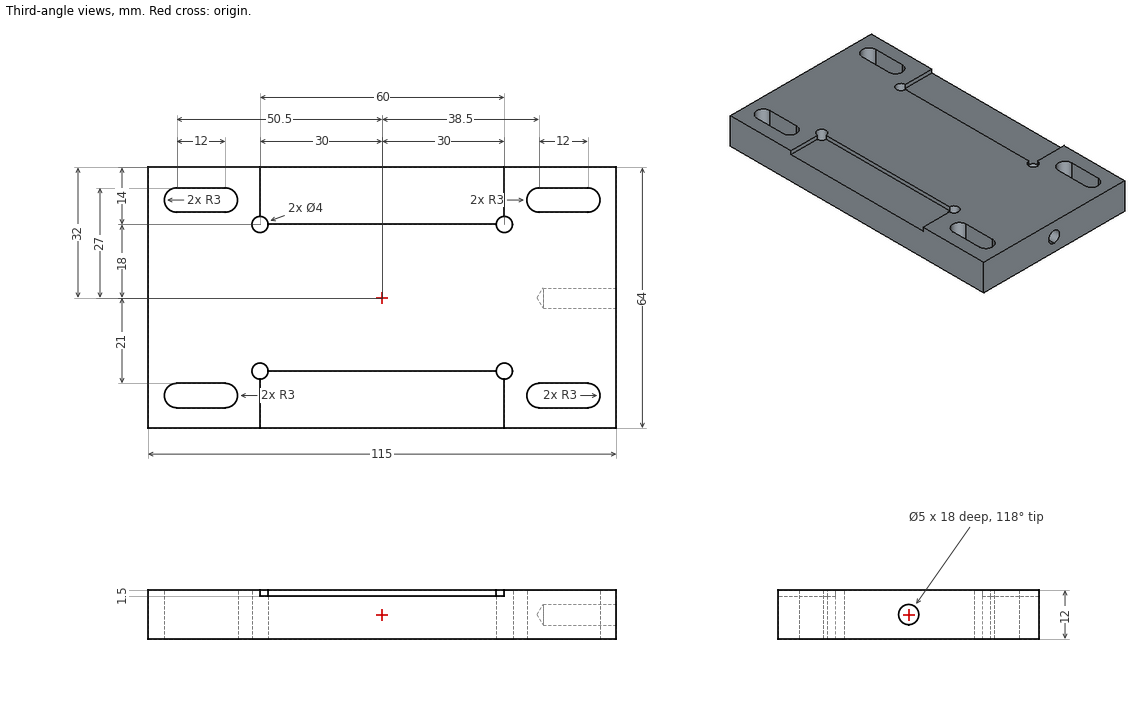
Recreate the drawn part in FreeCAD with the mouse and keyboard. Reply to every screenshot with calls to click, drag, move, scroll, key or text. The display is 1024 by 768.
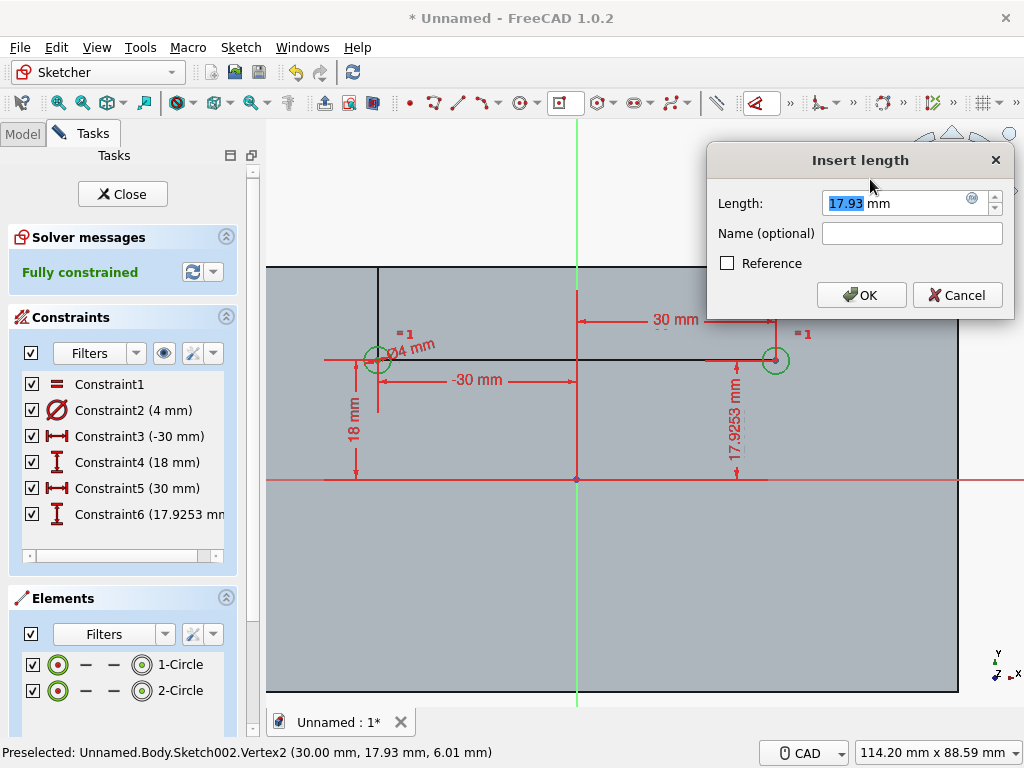
text(18)
key(Return)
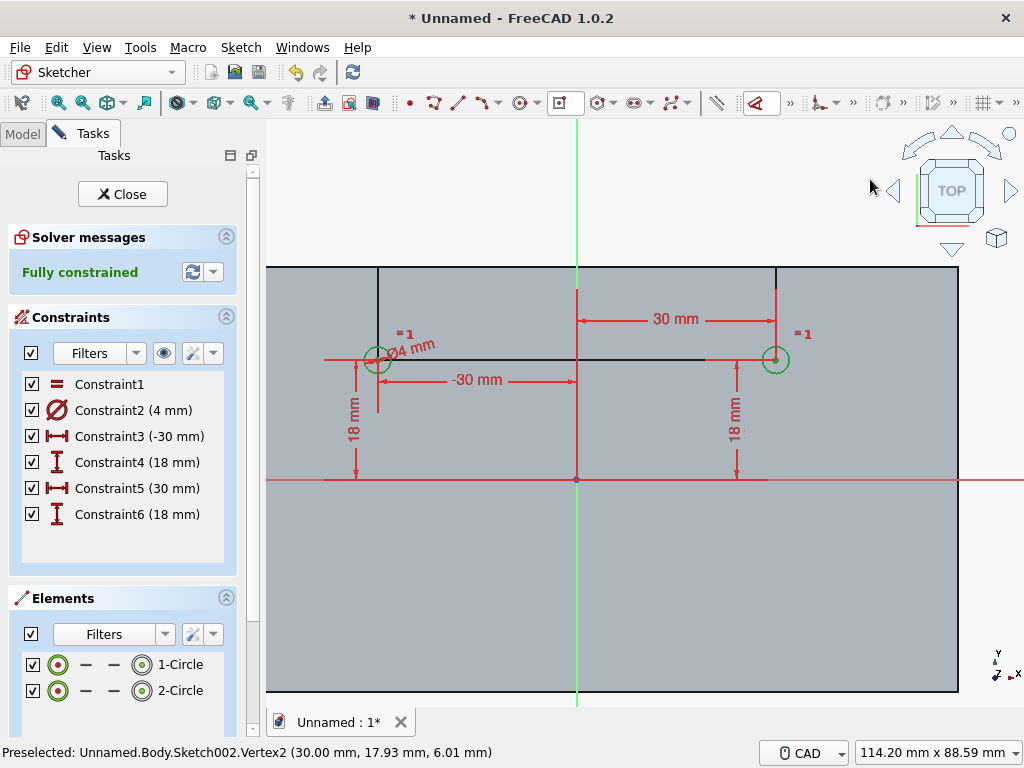
click(123, 194)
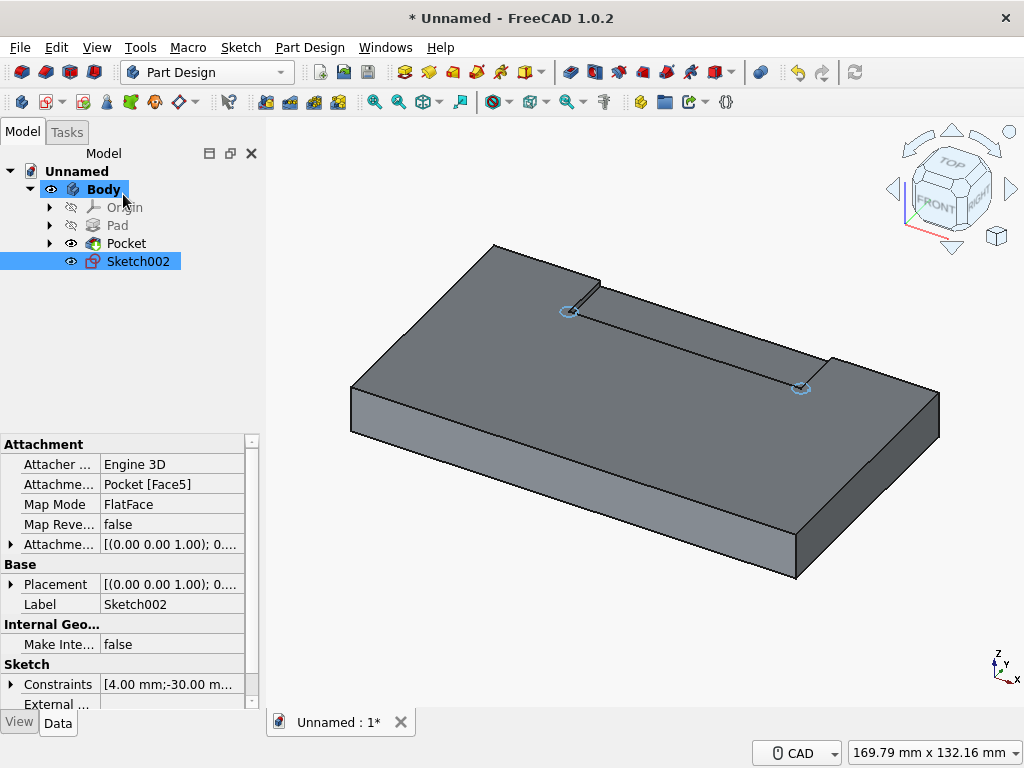
click(572, 72)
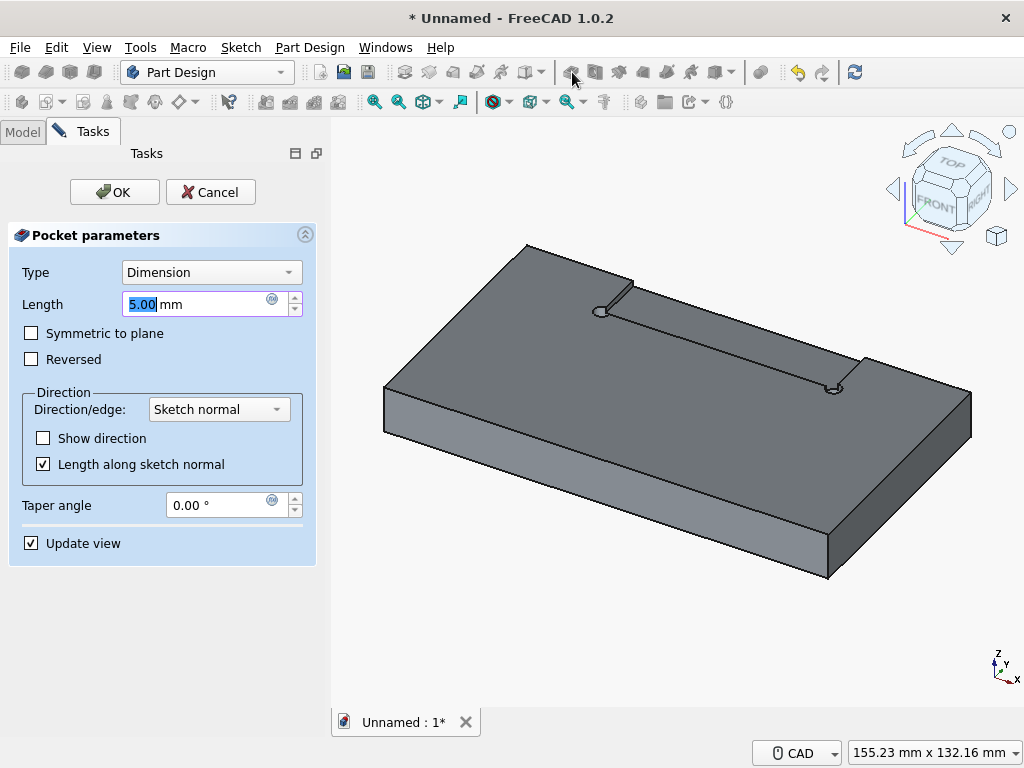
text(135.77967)
key(Tab)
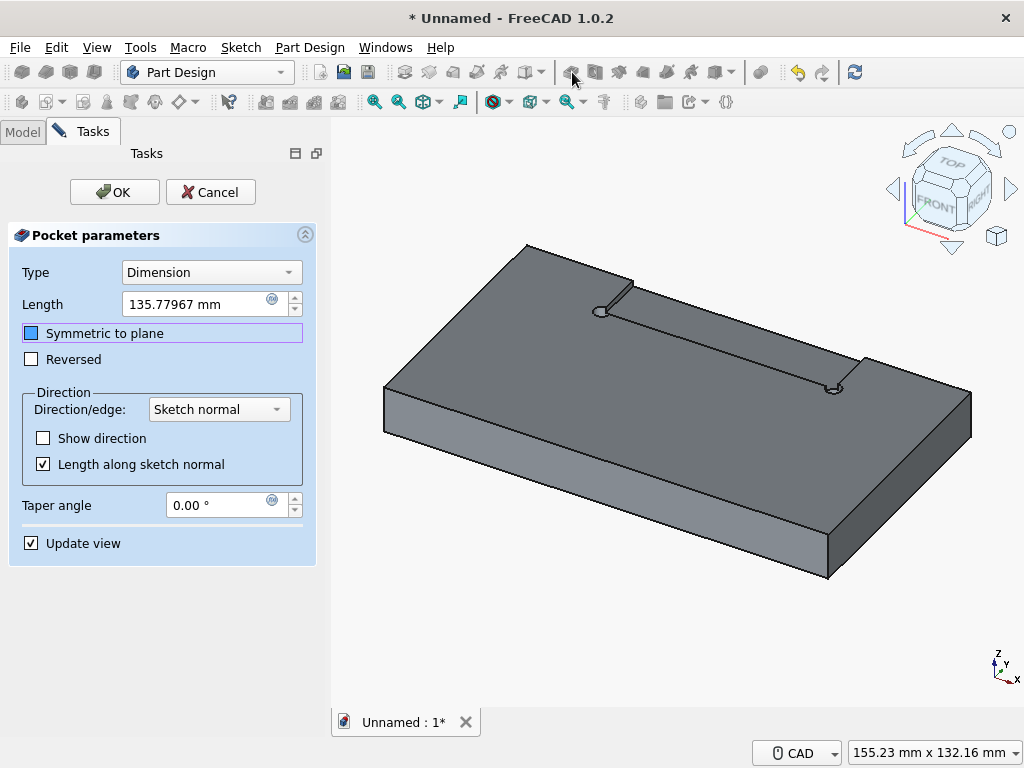
click(30, 333)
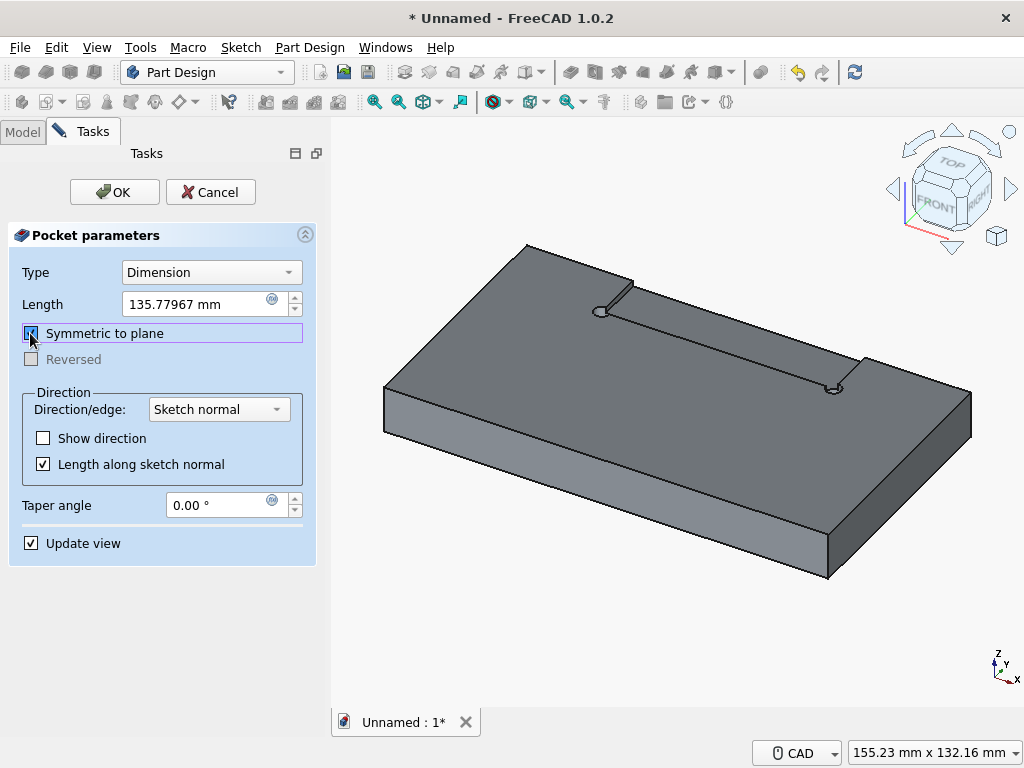
click(115, 192)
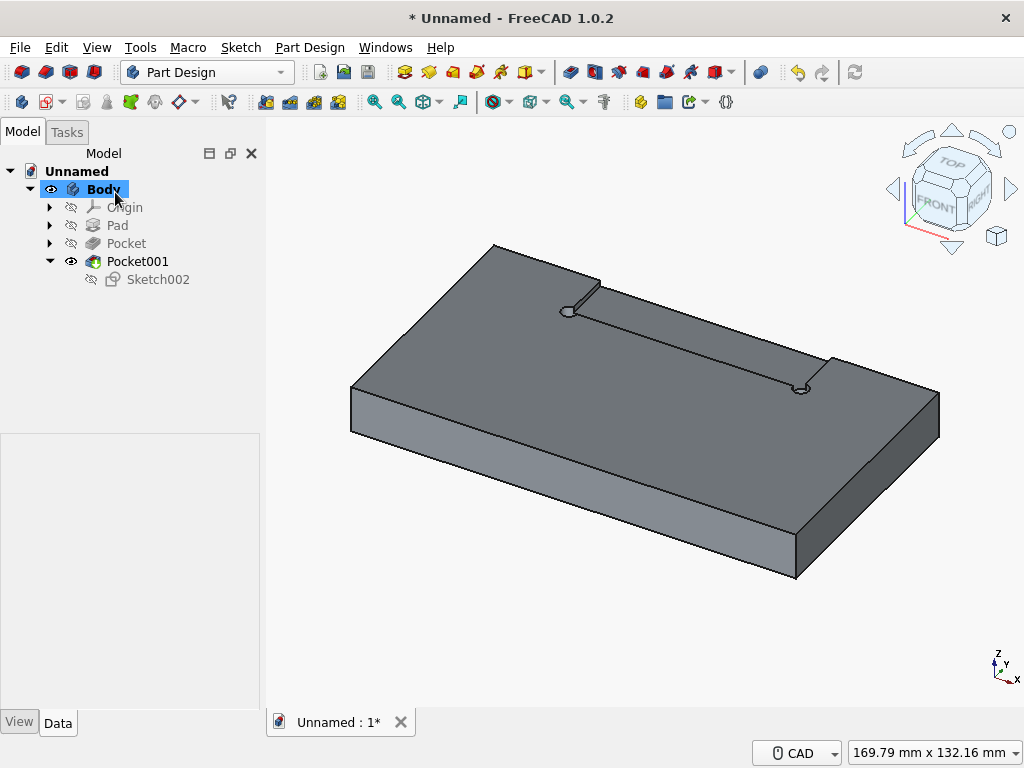
click(116, 243)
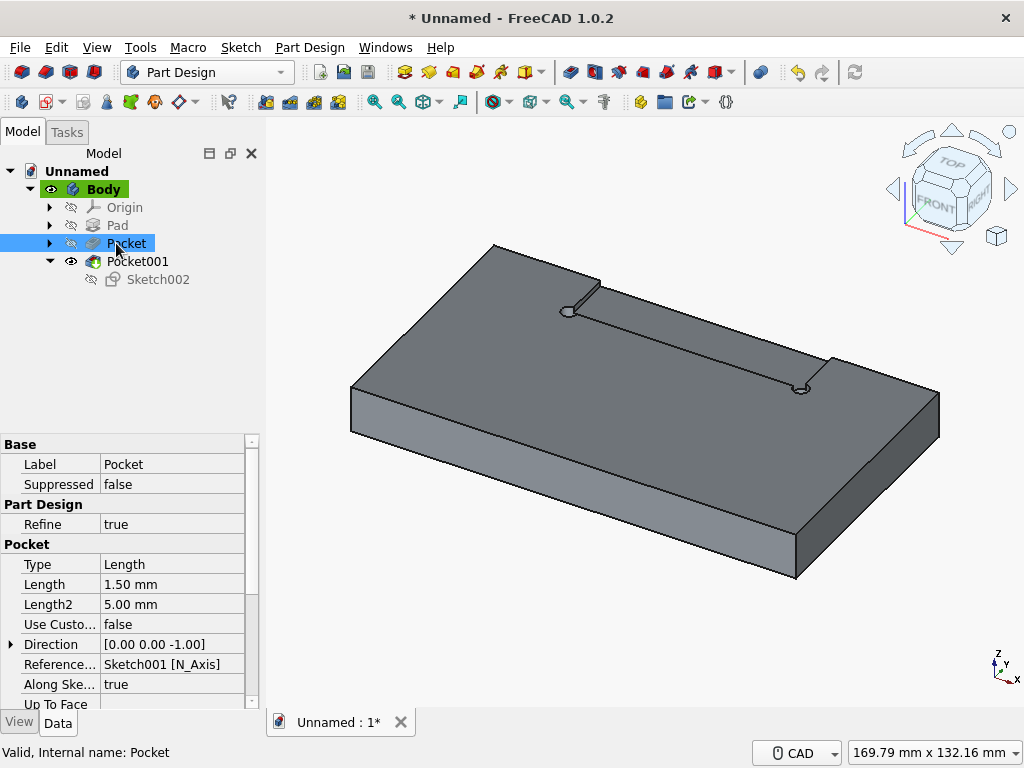
click(116, 261, ctrl)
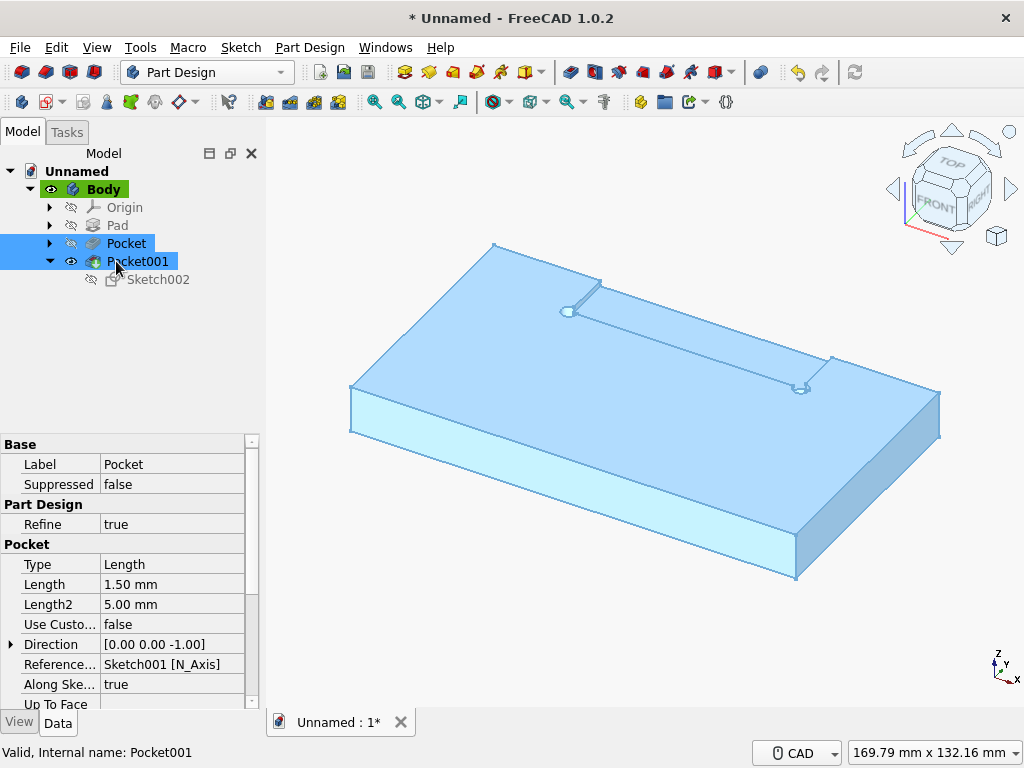
click(266, 102)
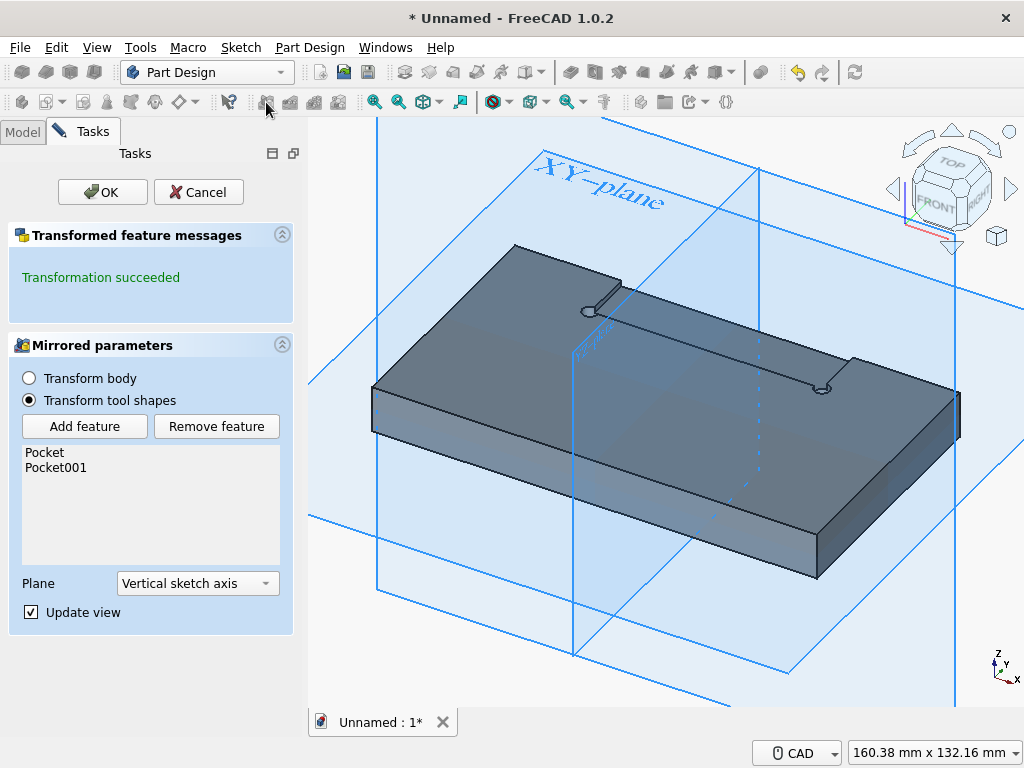
click(198, 584)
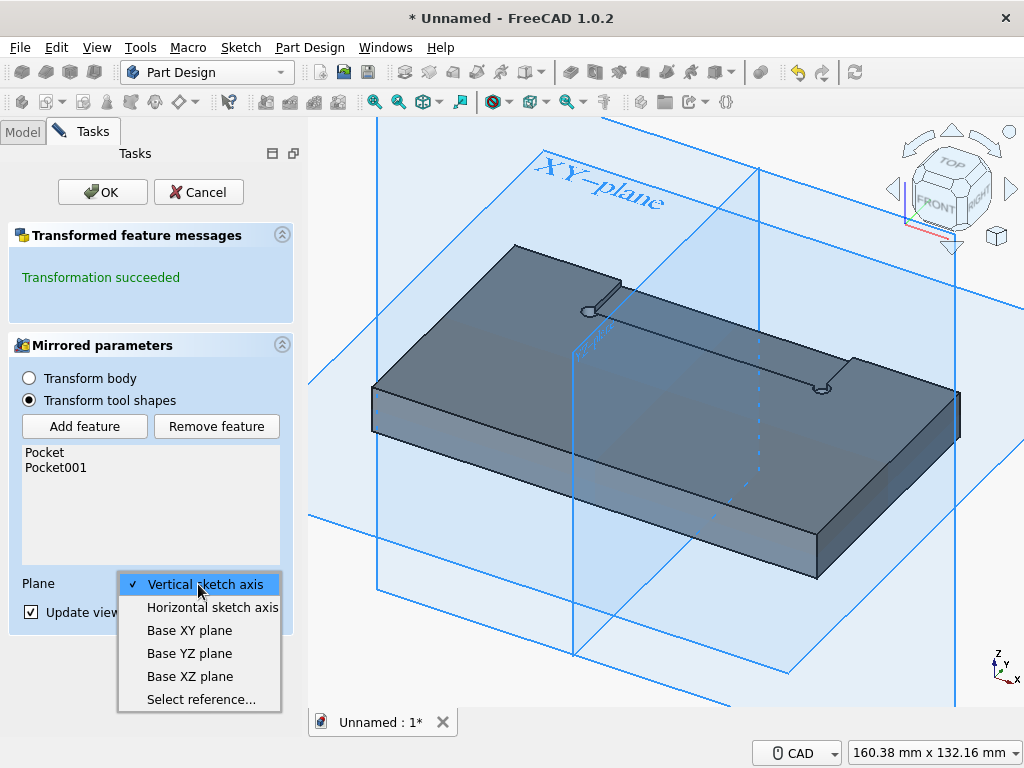
click(198, 676)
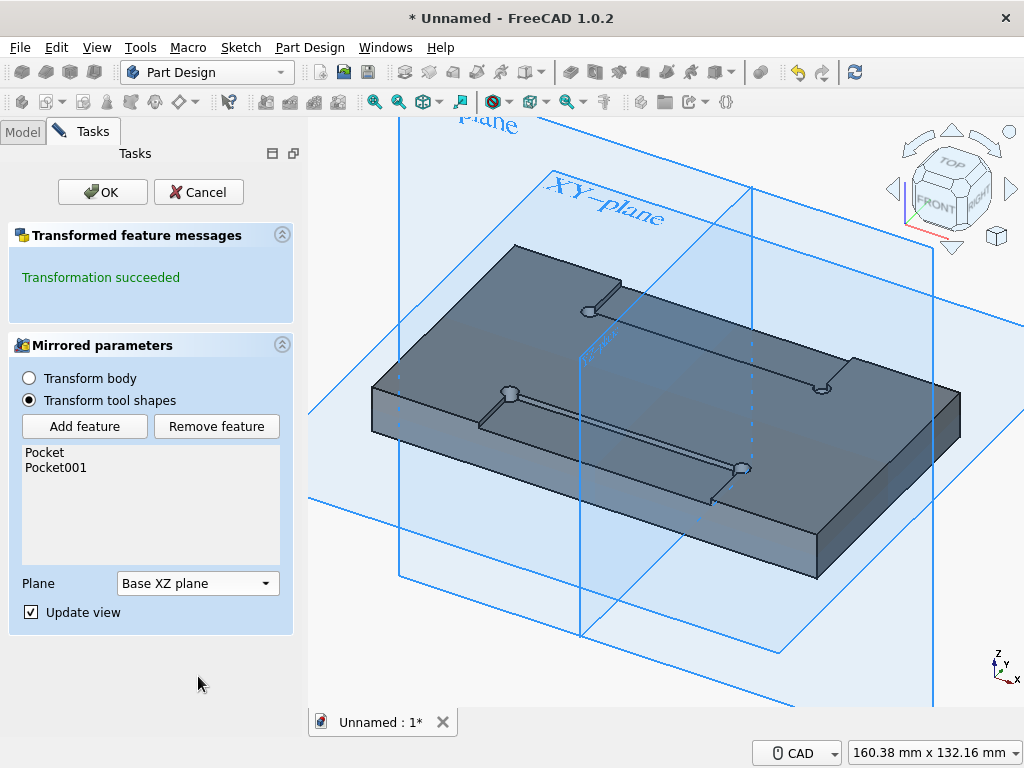
click(103, 192)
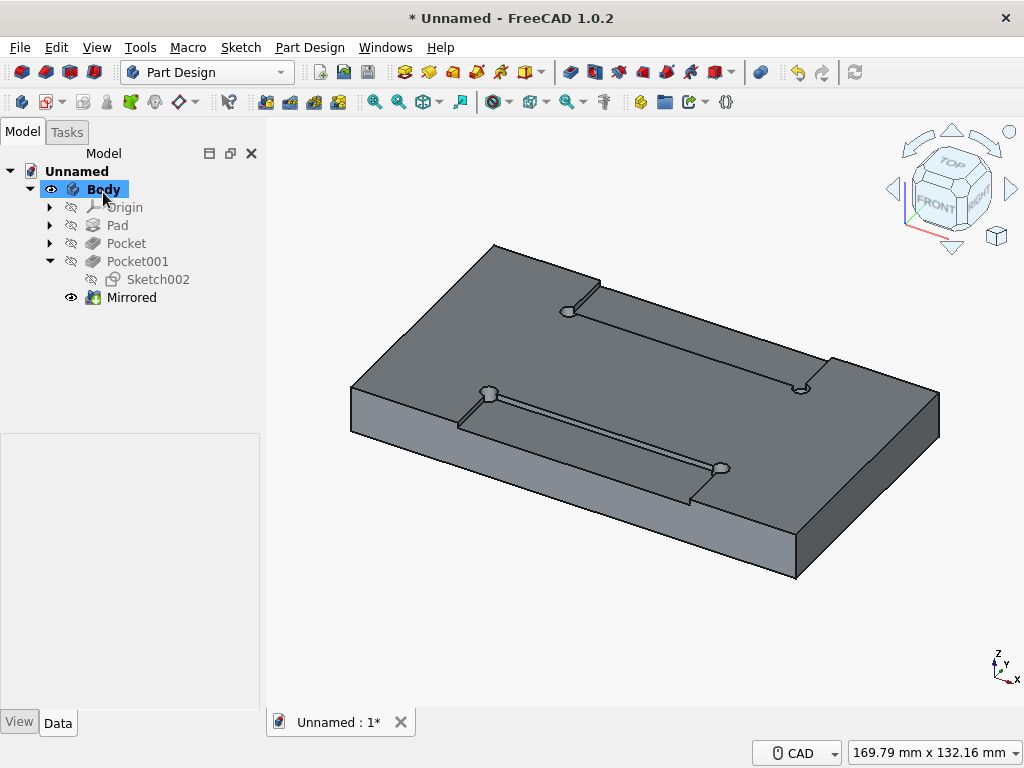
click(709, 410)